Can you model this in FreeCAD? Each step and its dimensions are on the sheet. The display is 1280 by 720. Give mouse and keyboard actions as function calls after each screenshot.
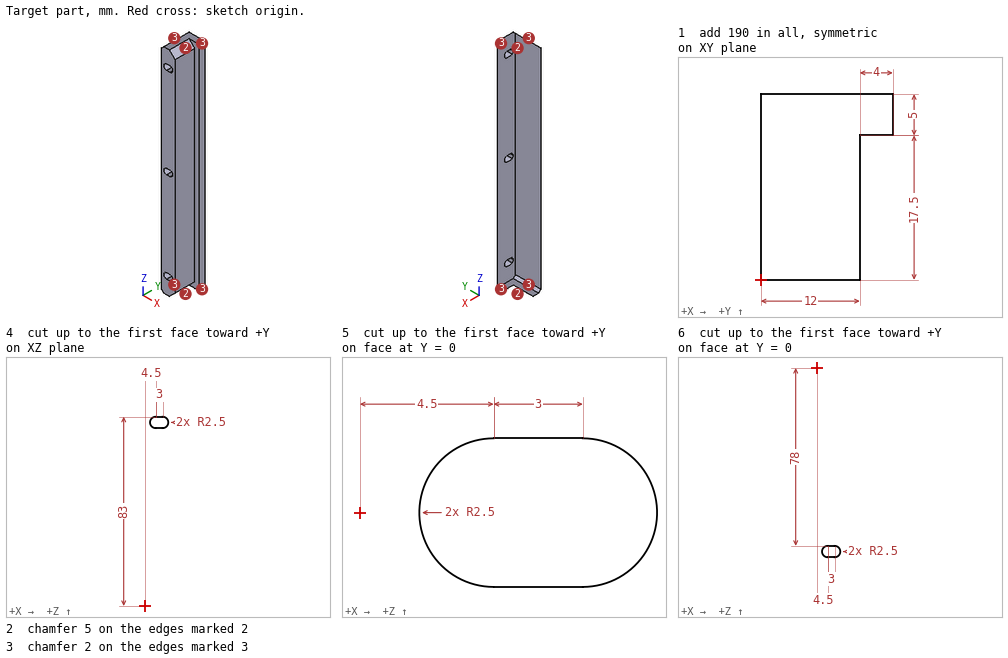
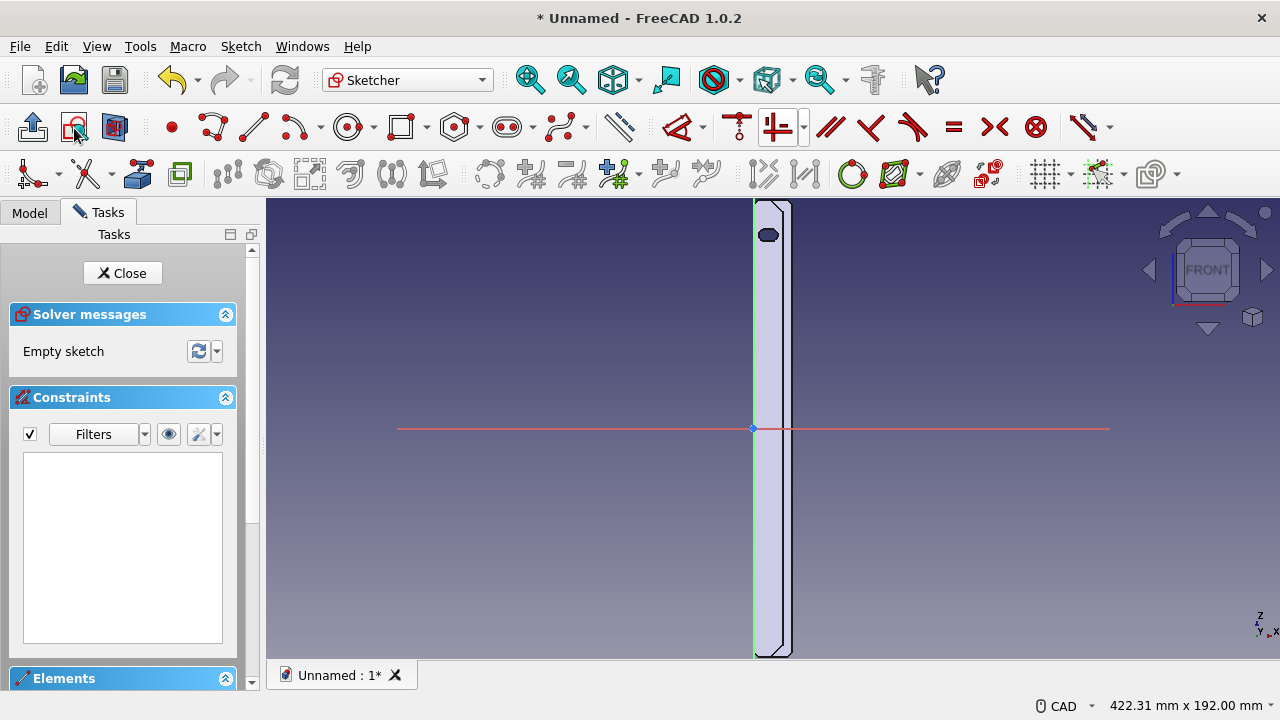
scroll(769, 428, up, 15)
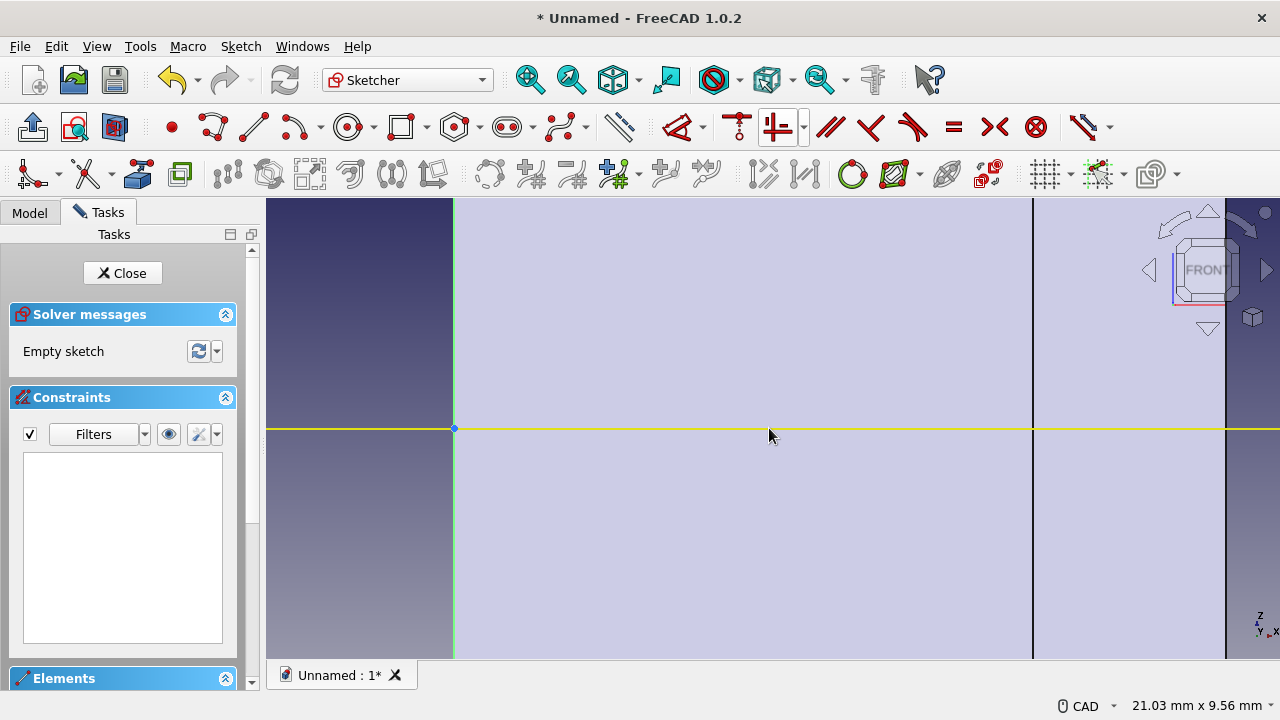
click(506, 128)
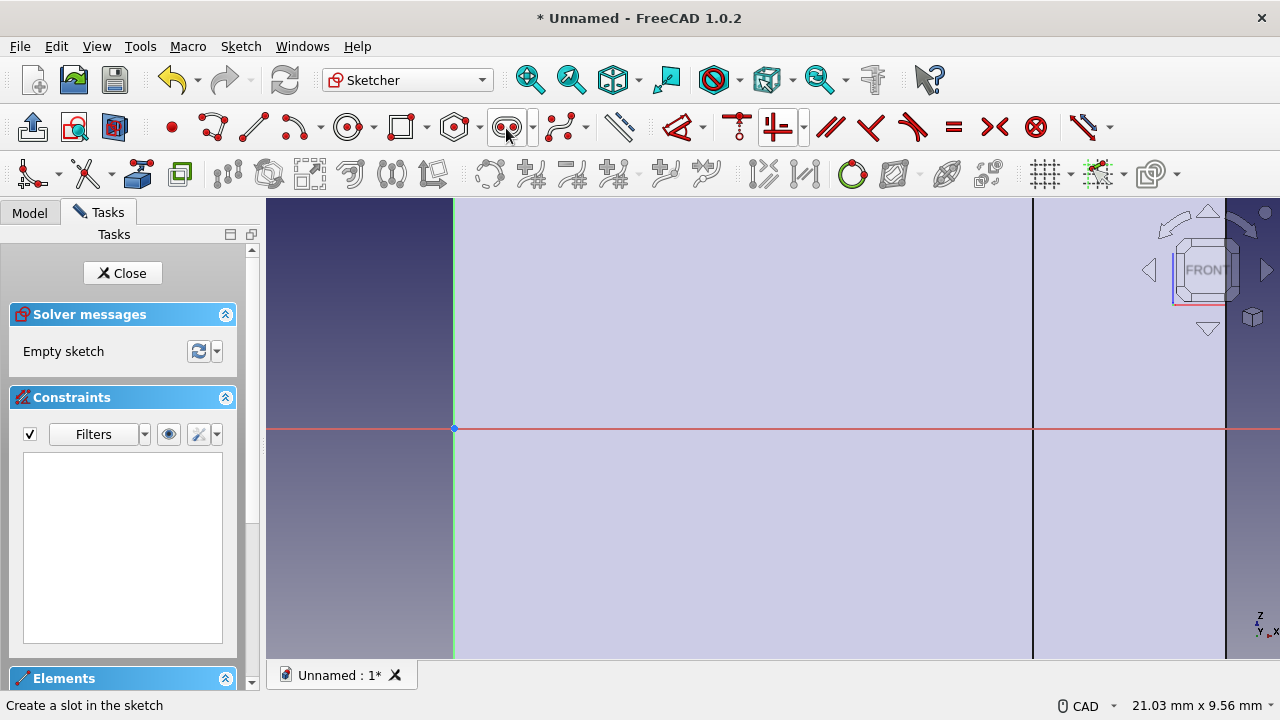
click(671, 428)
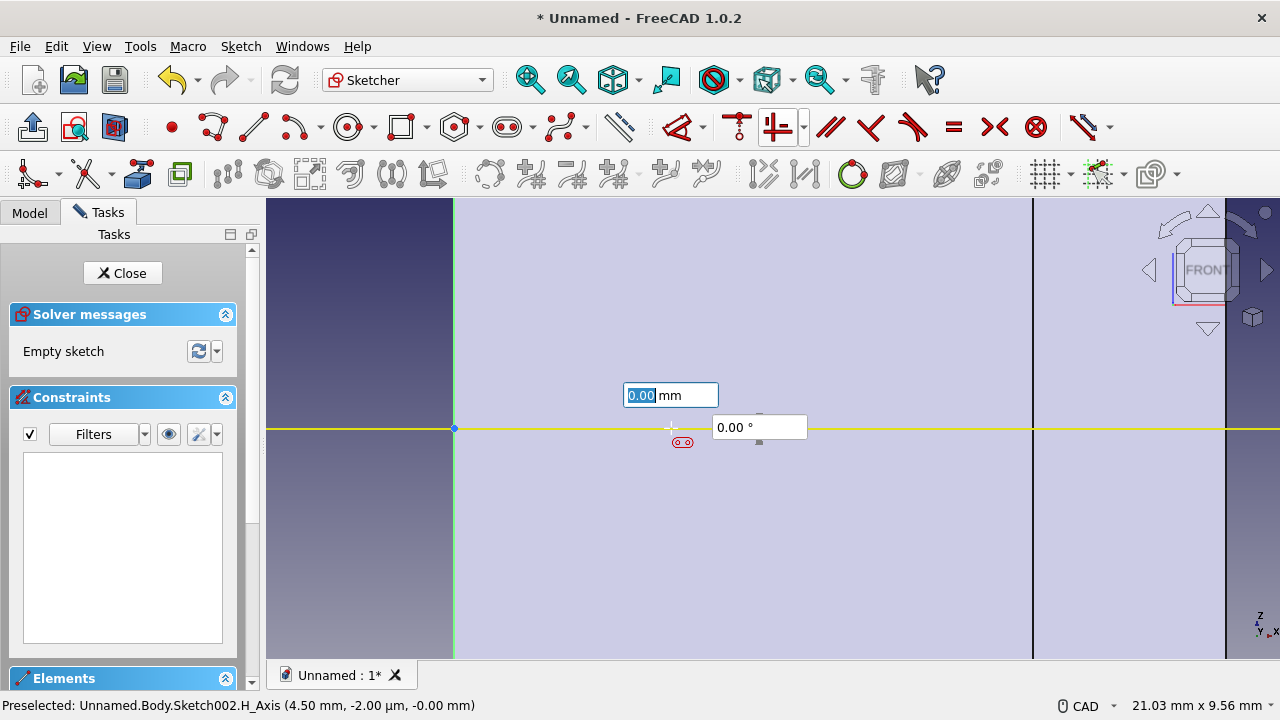
click(816, 419)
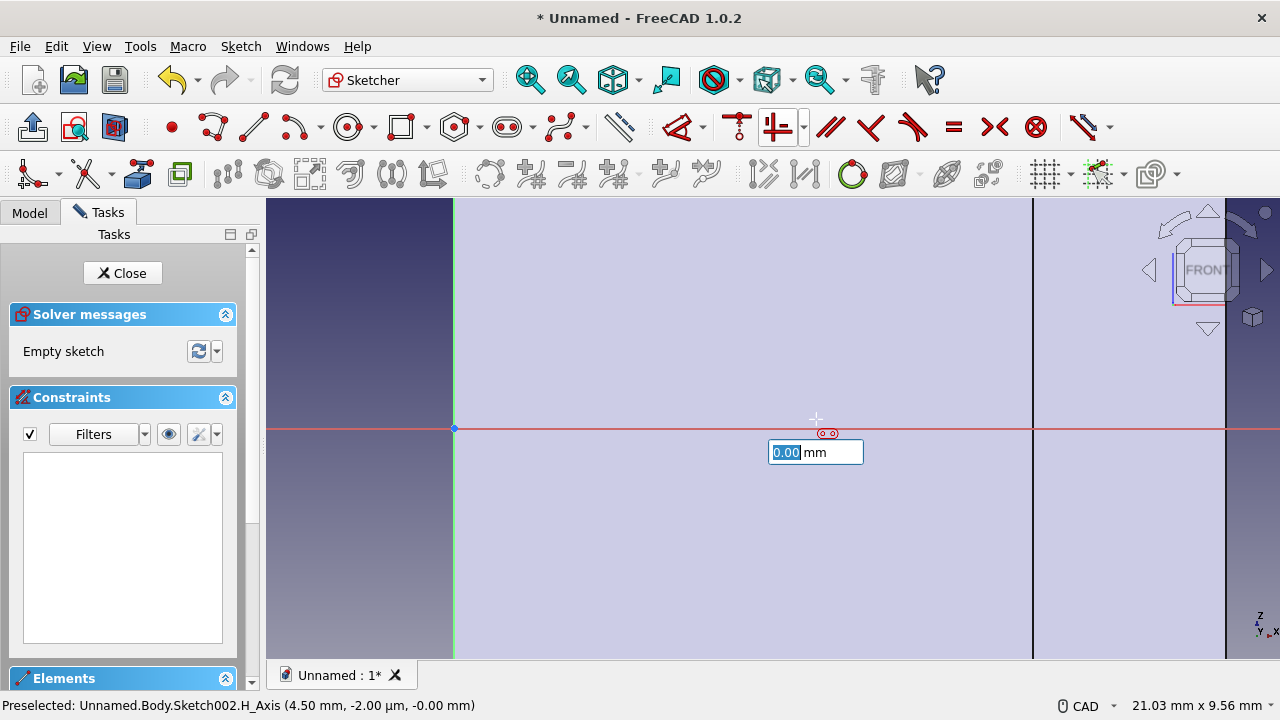
click(743, 308)
key(Escape)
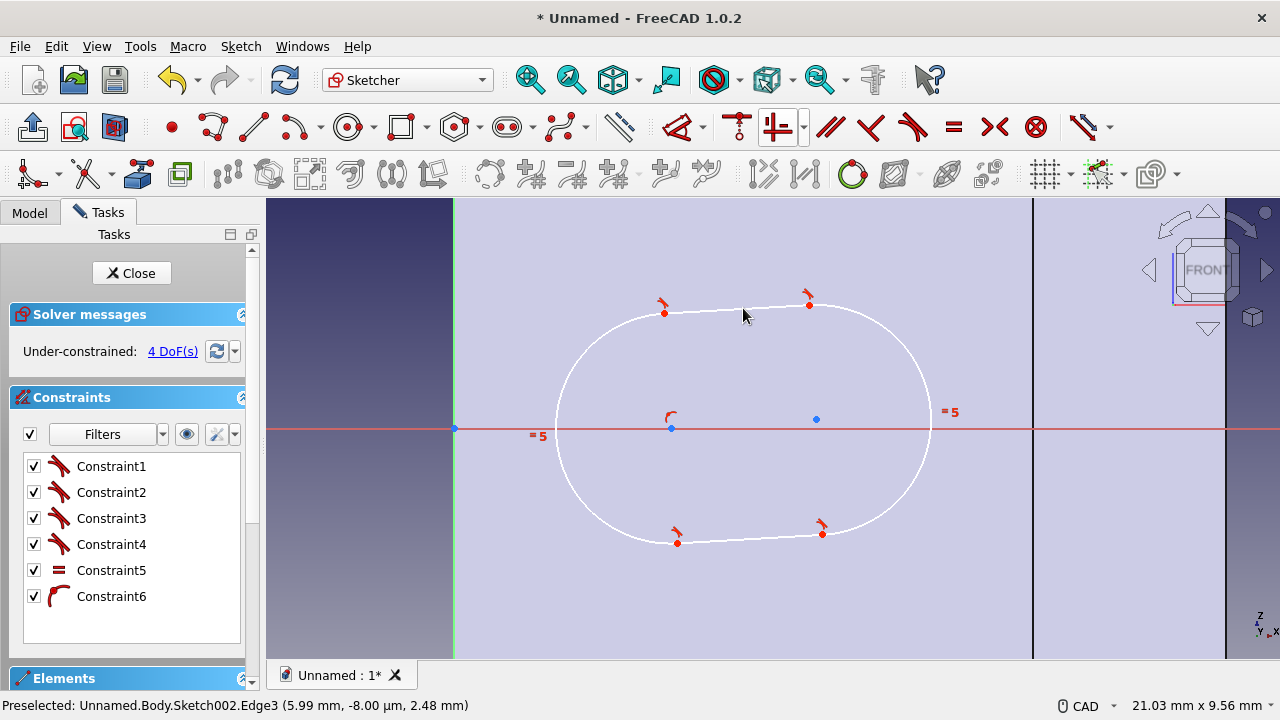
click(708, 311)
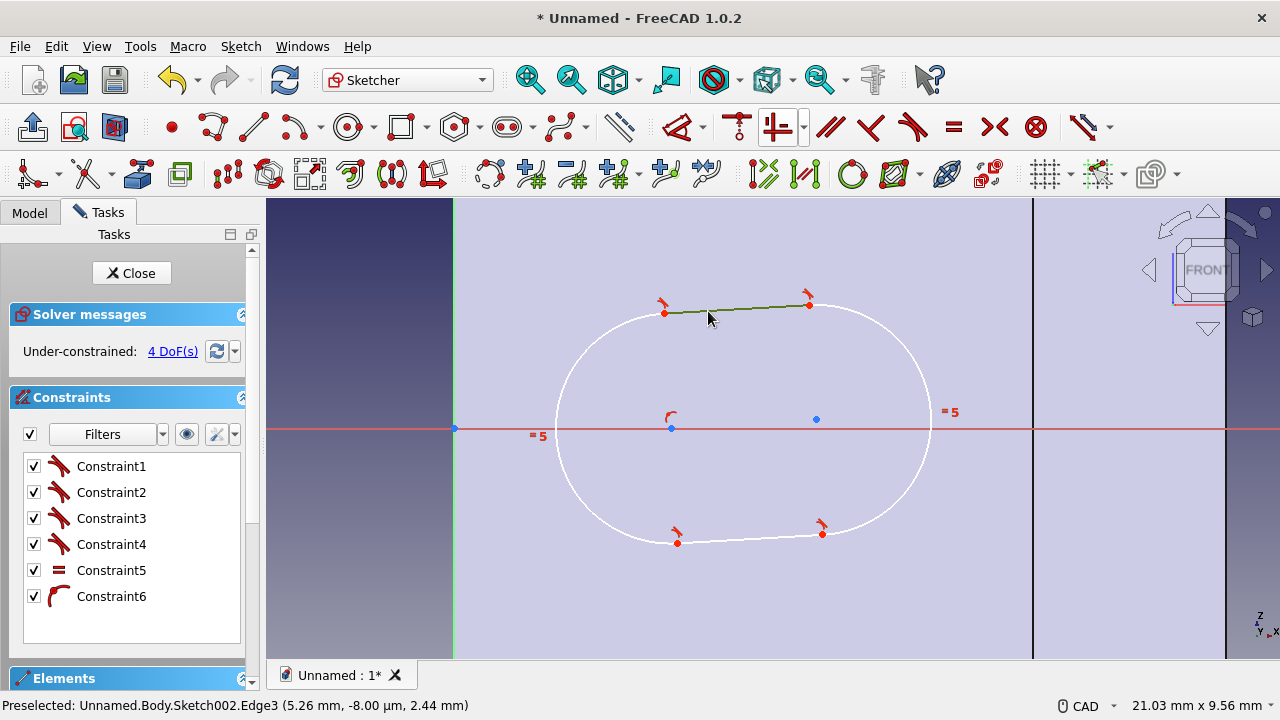
click(804, 128)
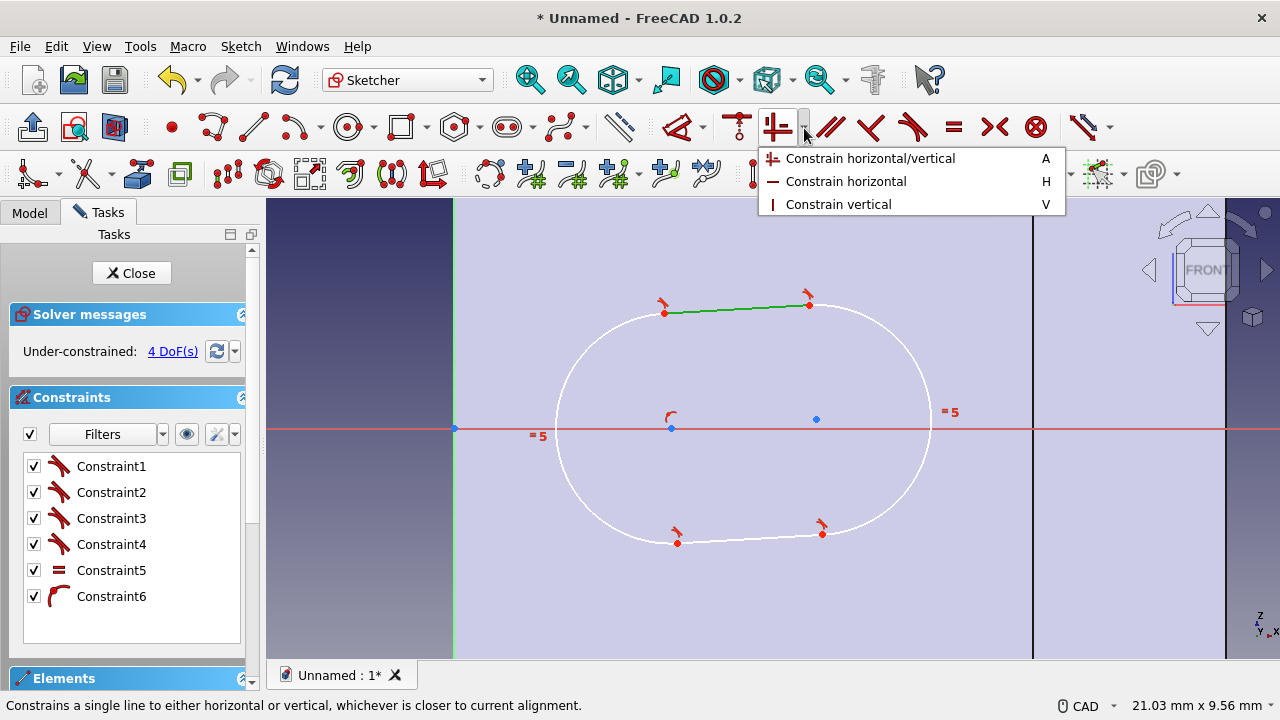
click(912, 182)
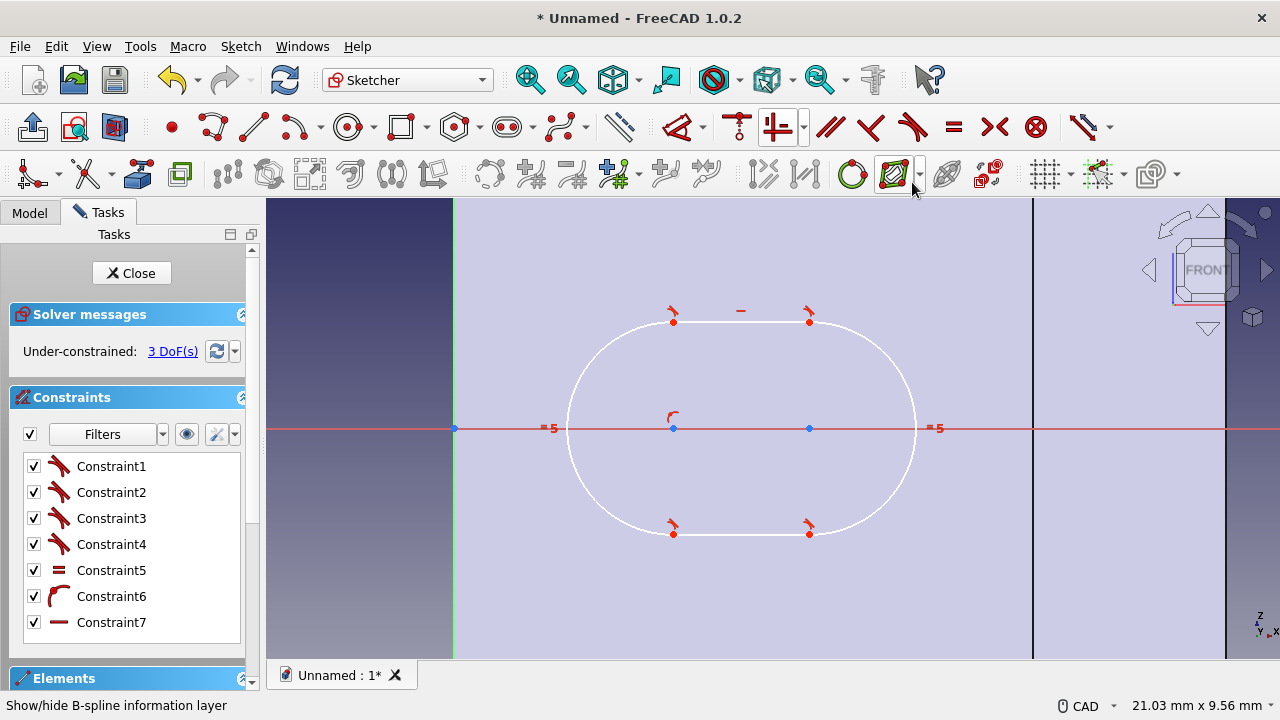
click(676, 128)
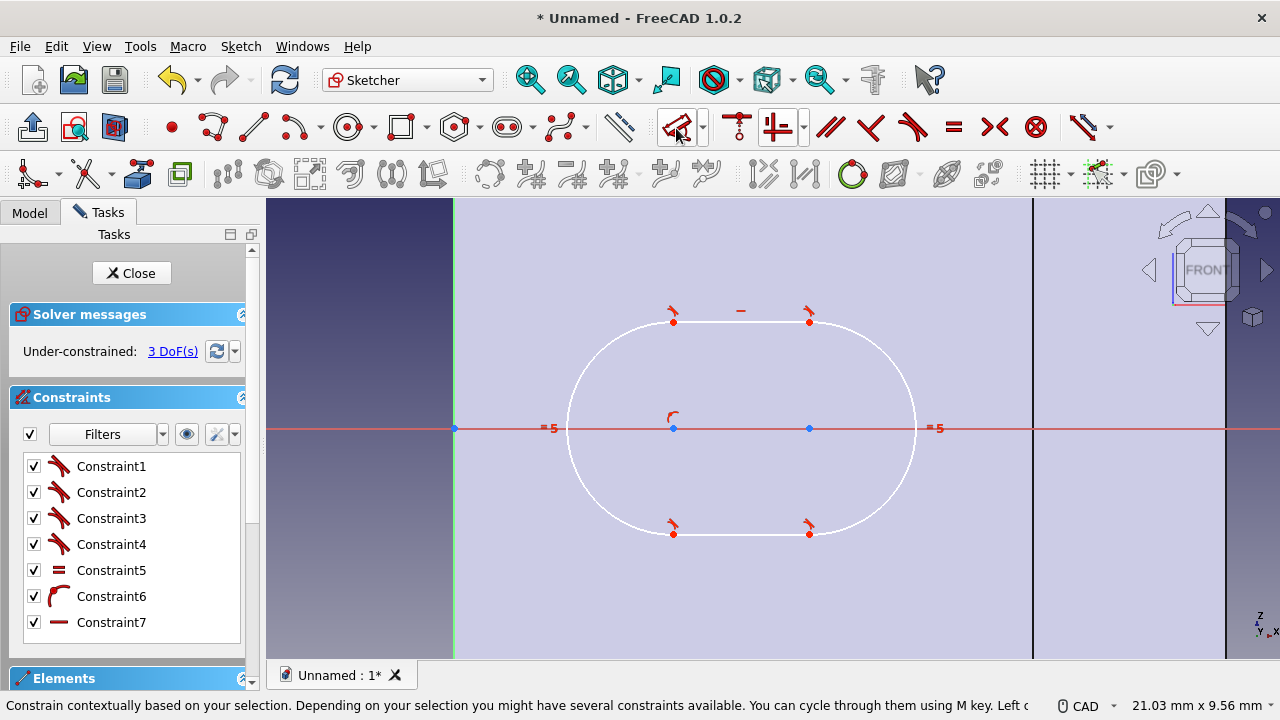
click(588, 366)
click(562, 347)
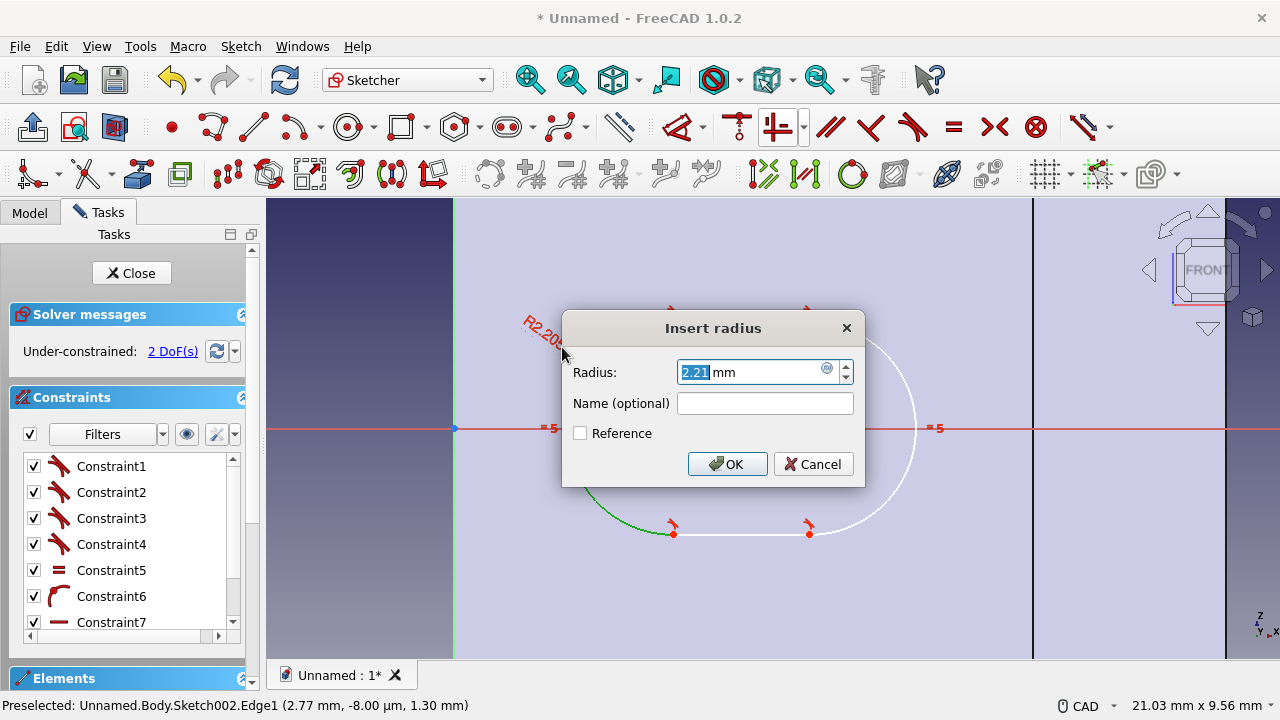
text(2.5)
key(Return)